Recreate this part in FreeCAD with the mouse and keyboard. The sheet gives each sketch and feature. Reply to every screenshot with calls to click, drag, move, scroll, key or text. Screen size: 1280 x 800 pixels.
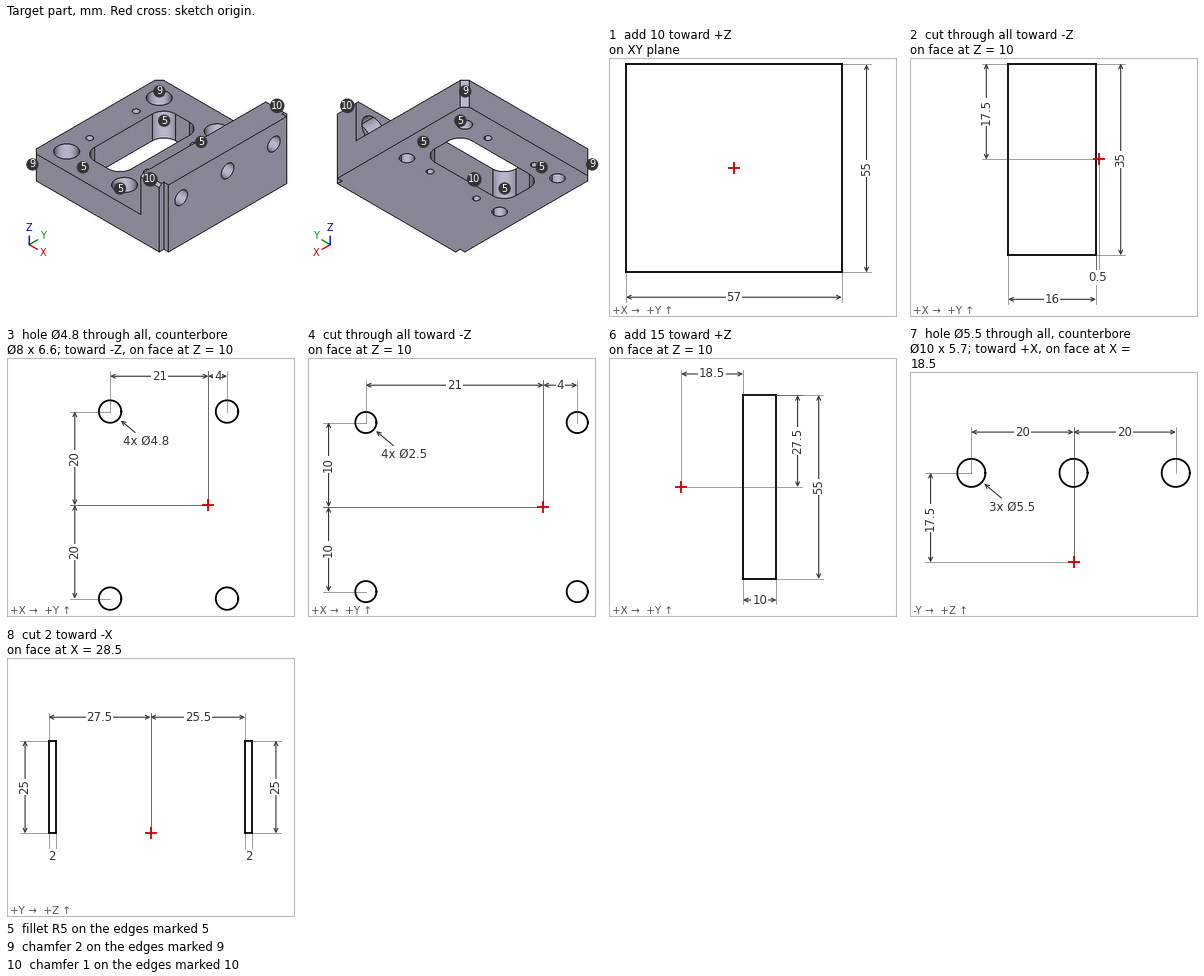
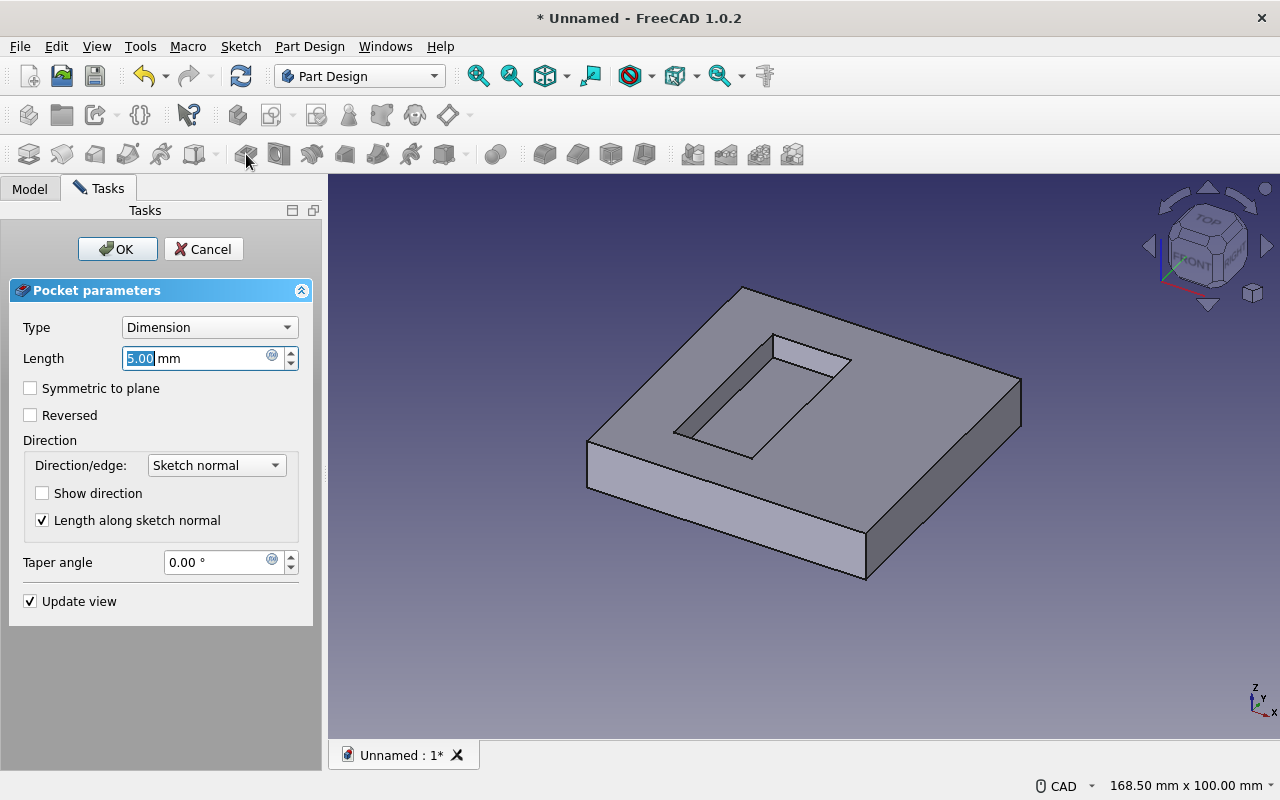
click(210, 328)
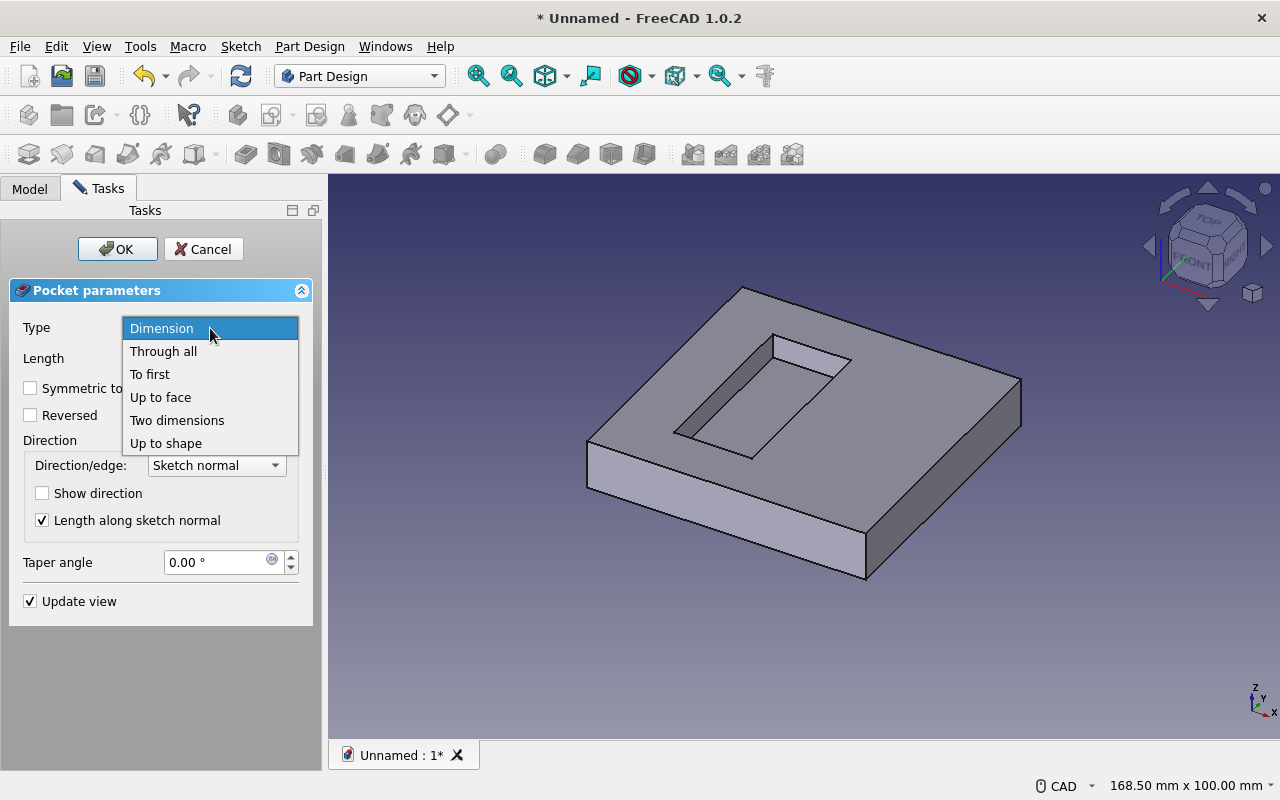
click(208, 352)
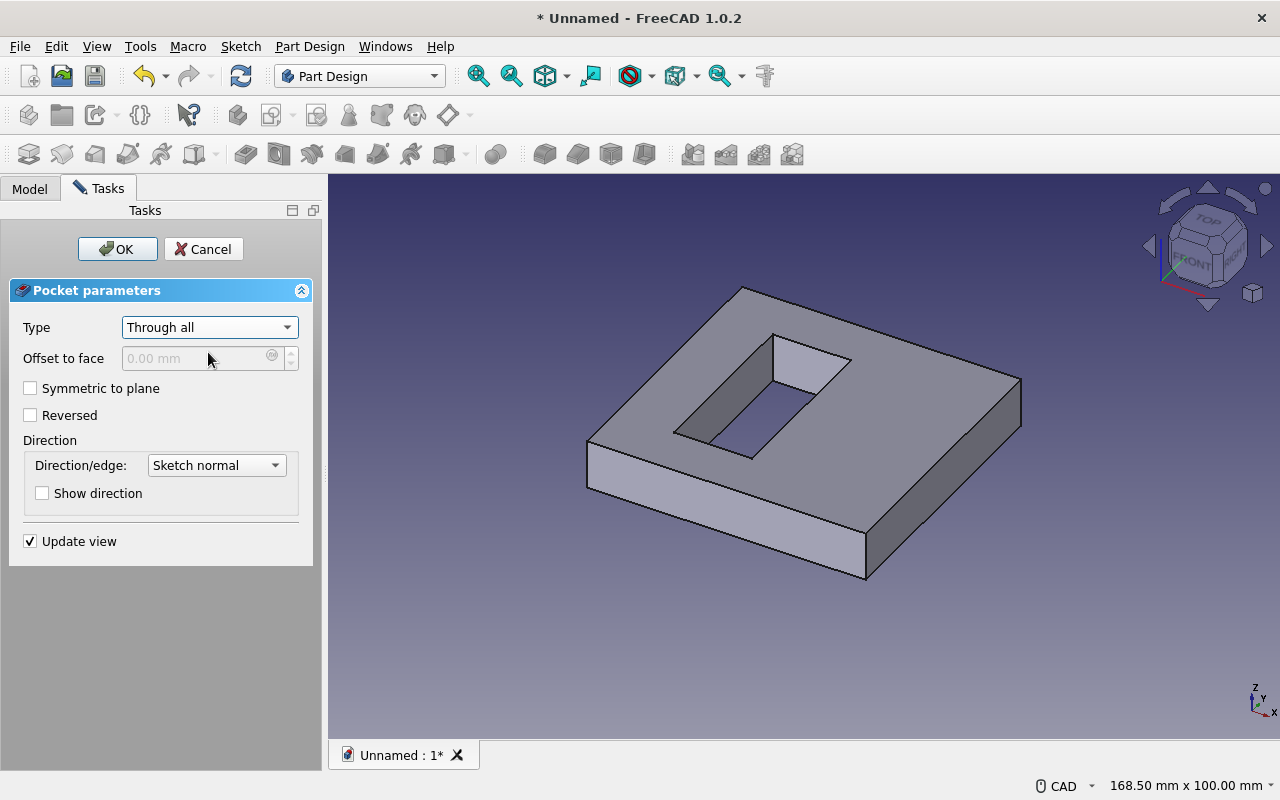
click(118, 249)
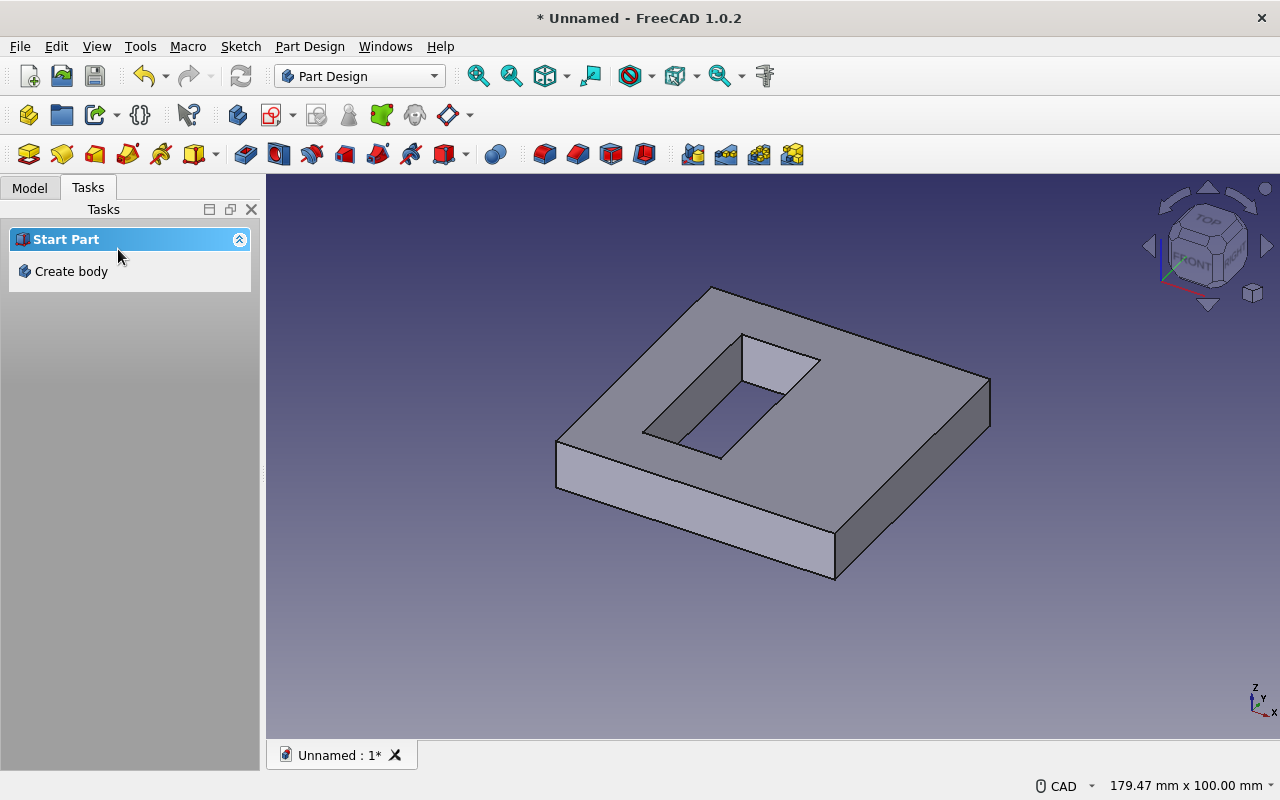
click(875, 414)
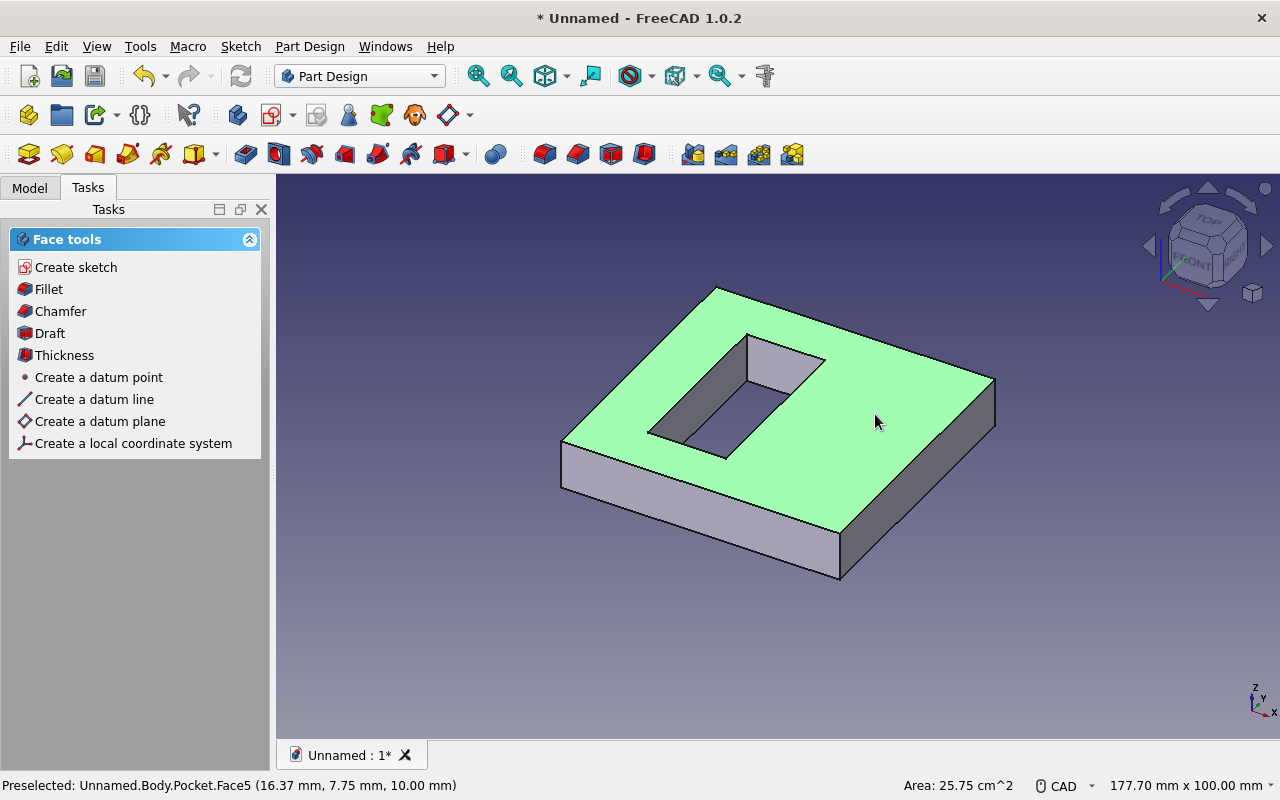
click(270, 116)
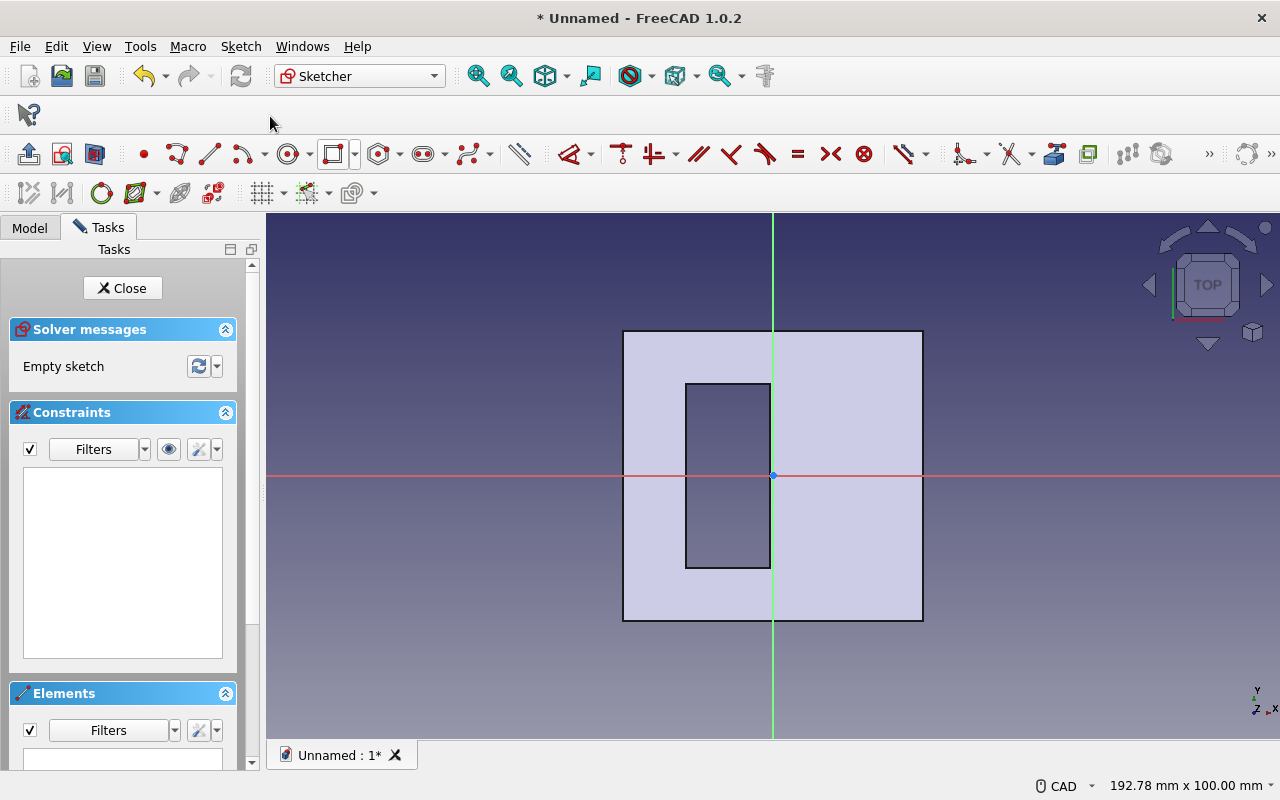
scroll(777, 476, up, 2)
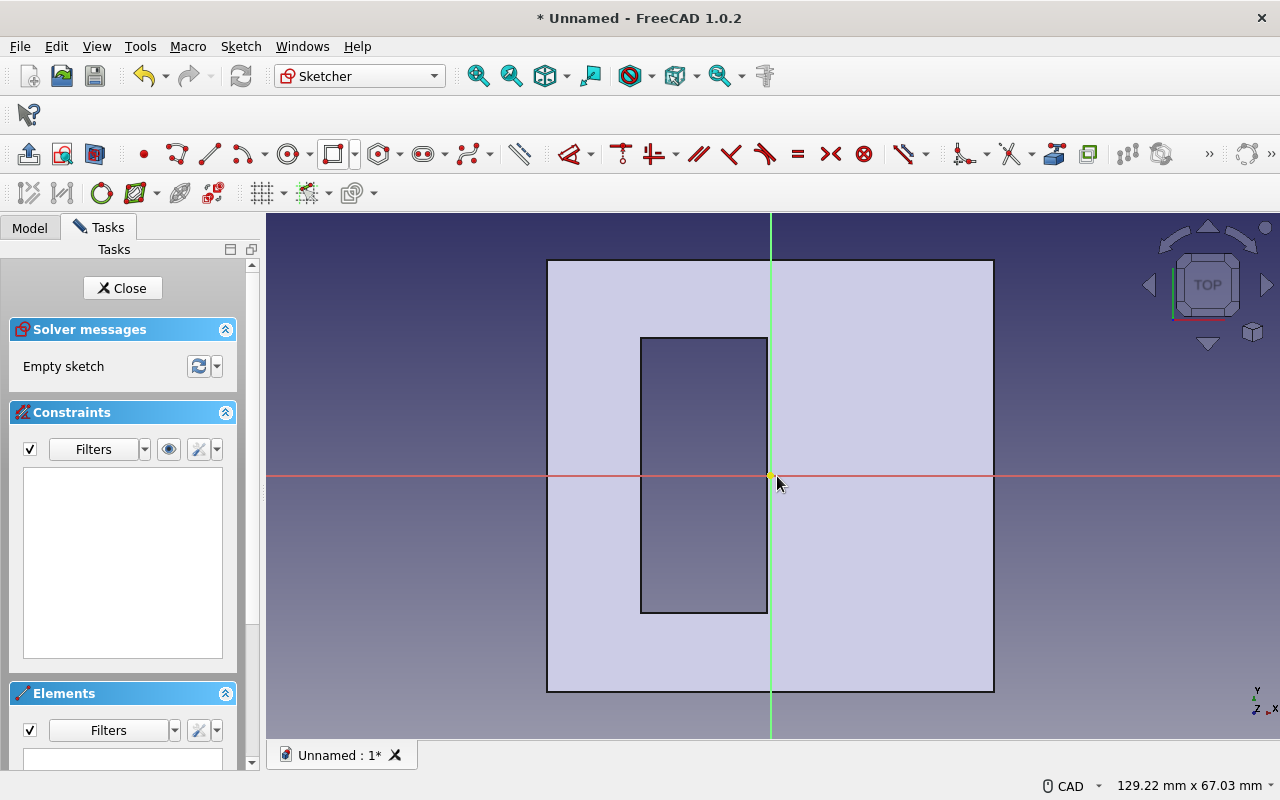
key(g)
key(c)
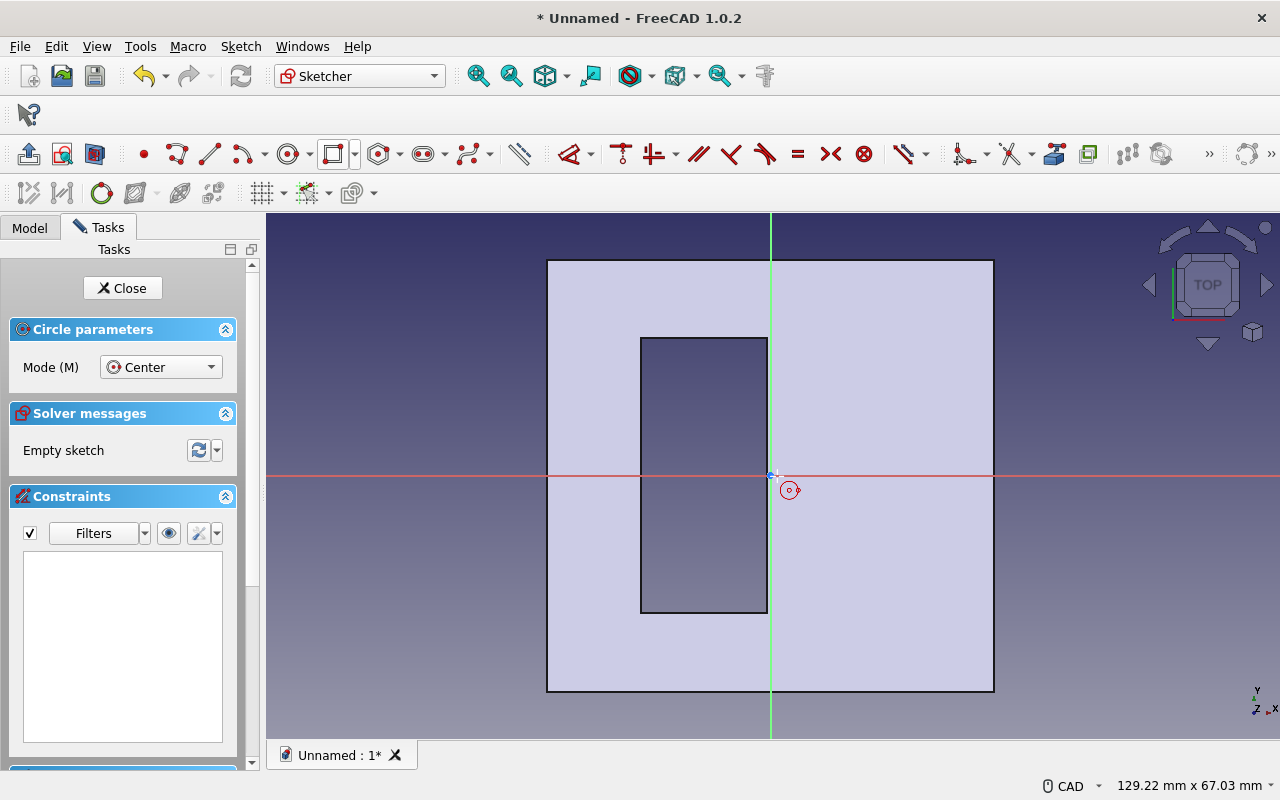
click(606, 319)
move(619, 305)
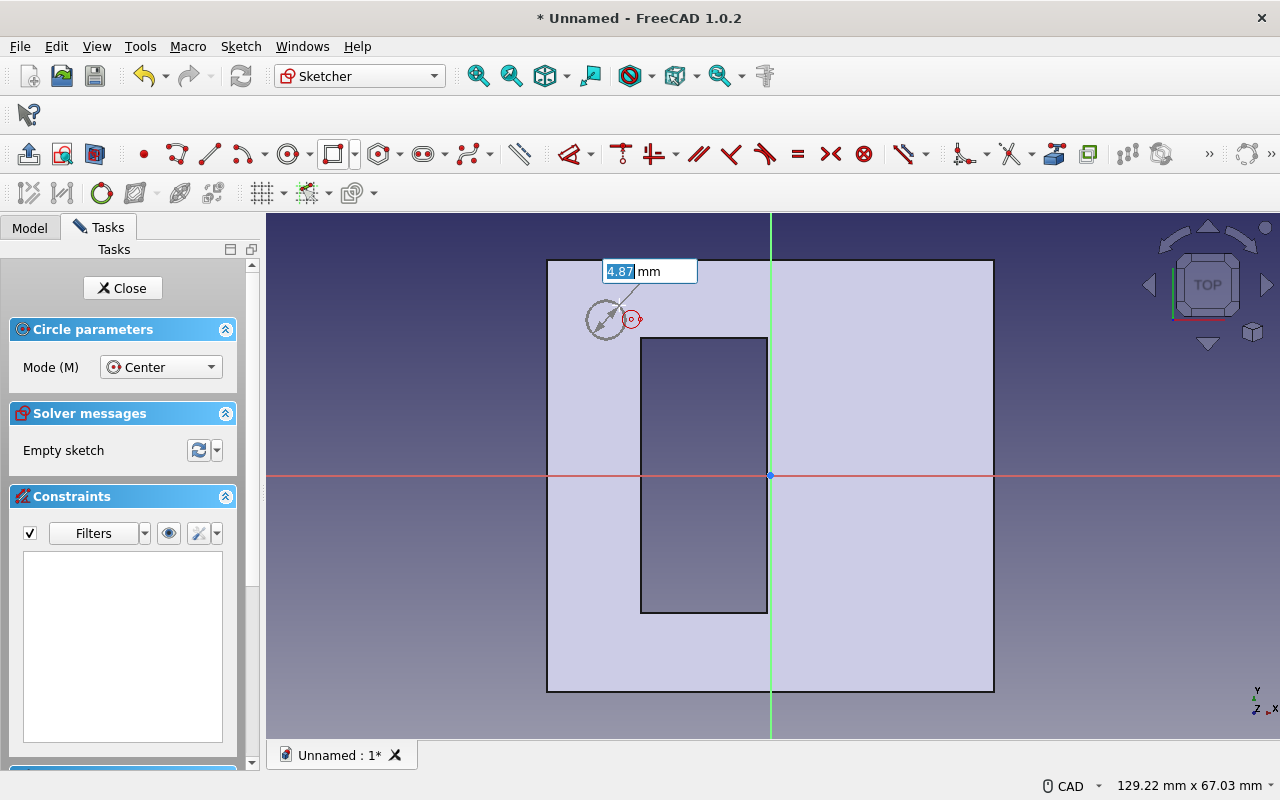
text(4.8)
key(Return)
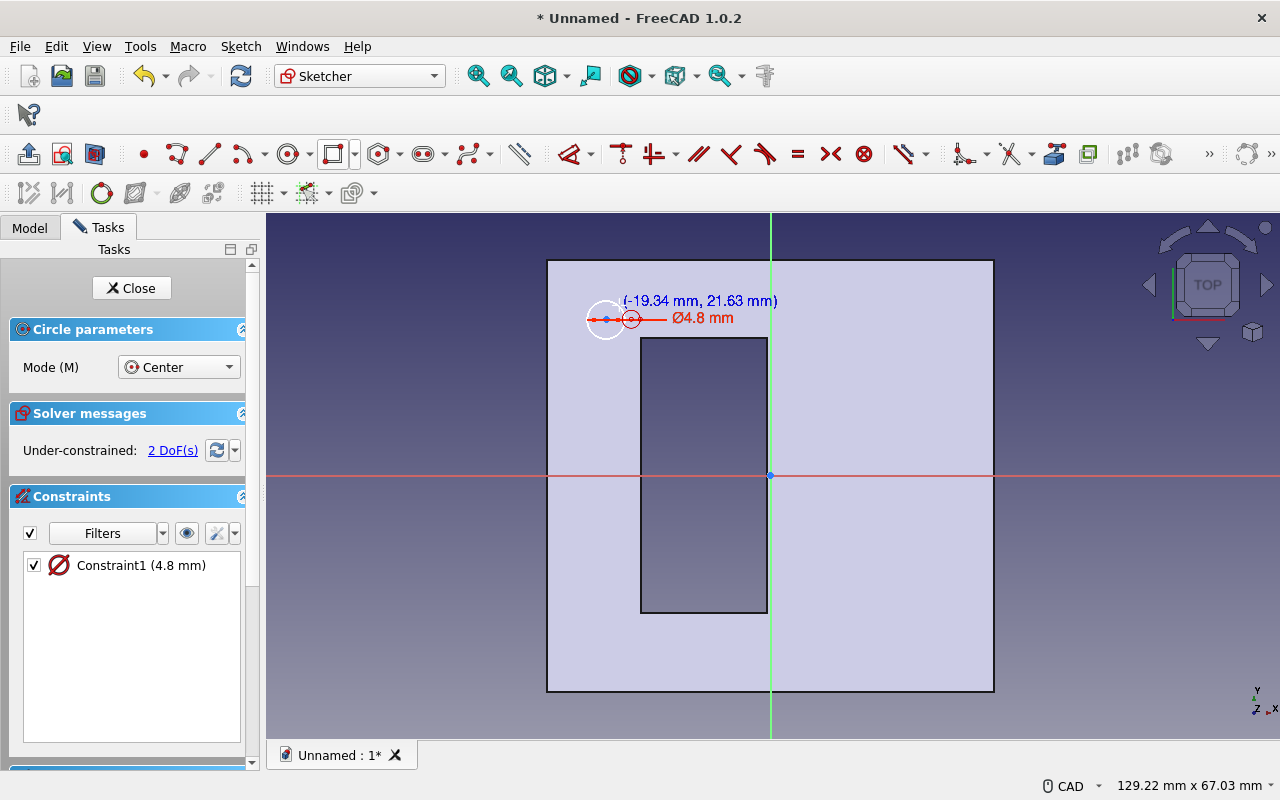
click(802, 319)
move(815, 305)